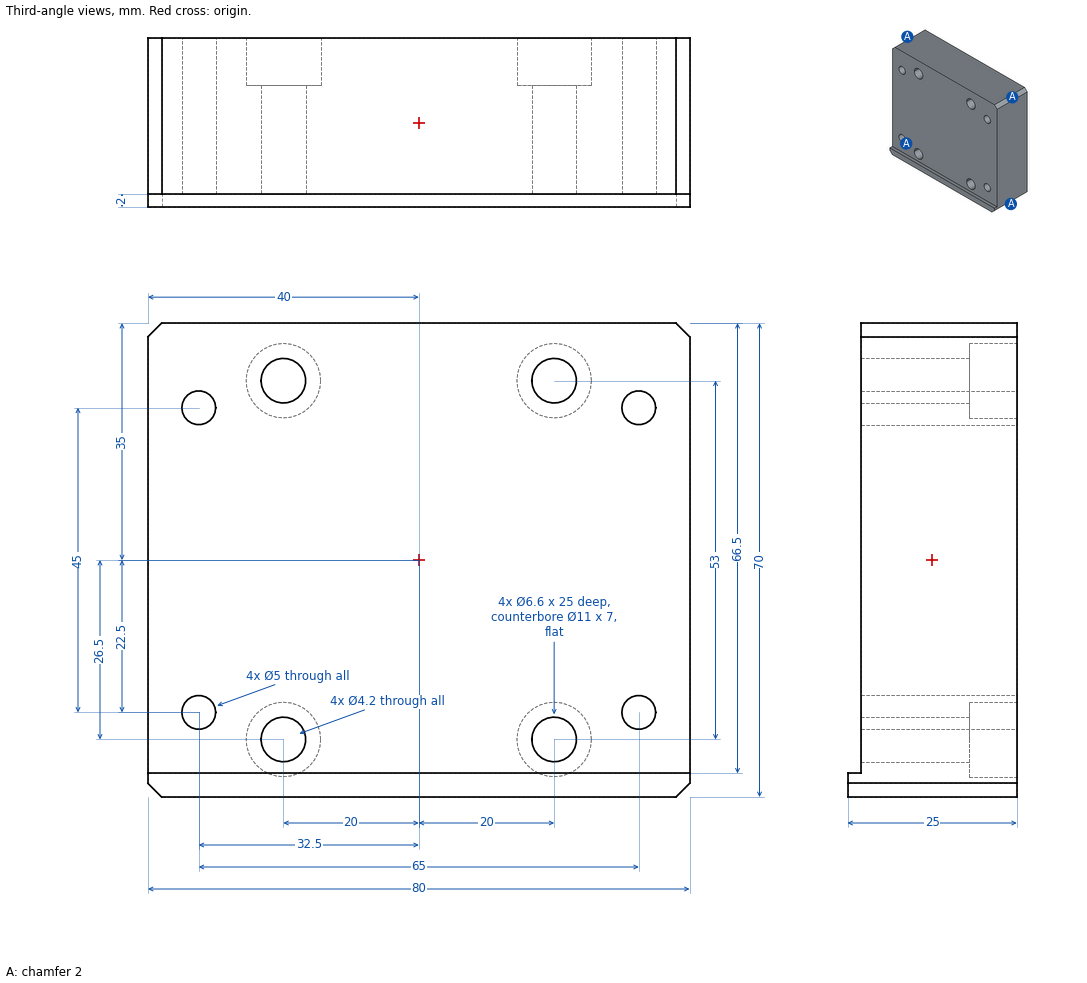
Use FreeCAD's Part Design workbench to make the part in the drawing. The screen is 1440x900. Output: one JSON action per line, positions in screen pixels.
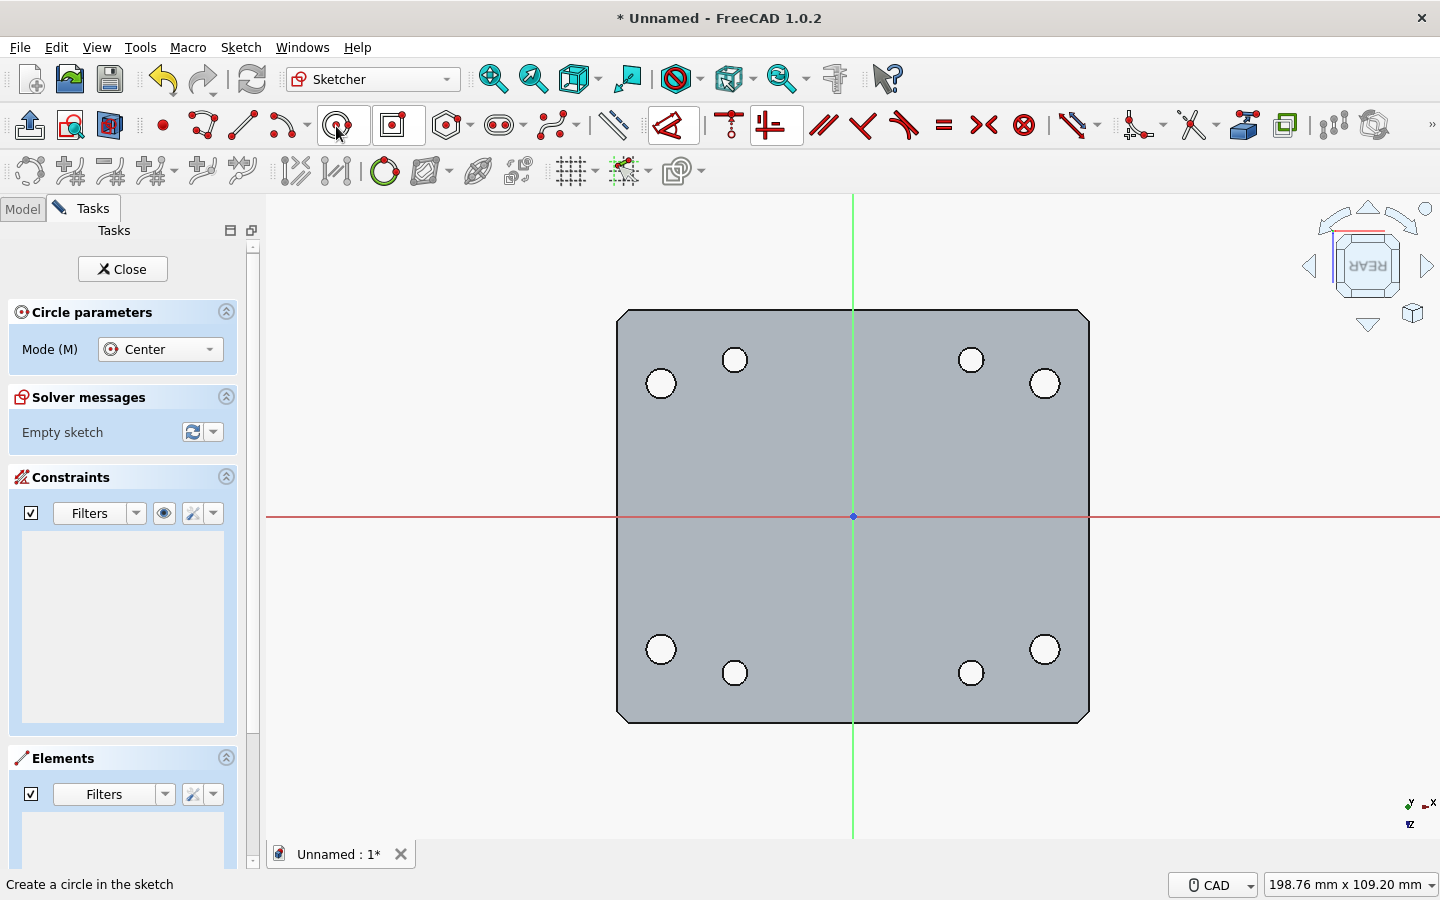
{"action": "left_click", "coordinate": [971, 360]}
{"action": "mouse_move", "coordinate": [985, 346]}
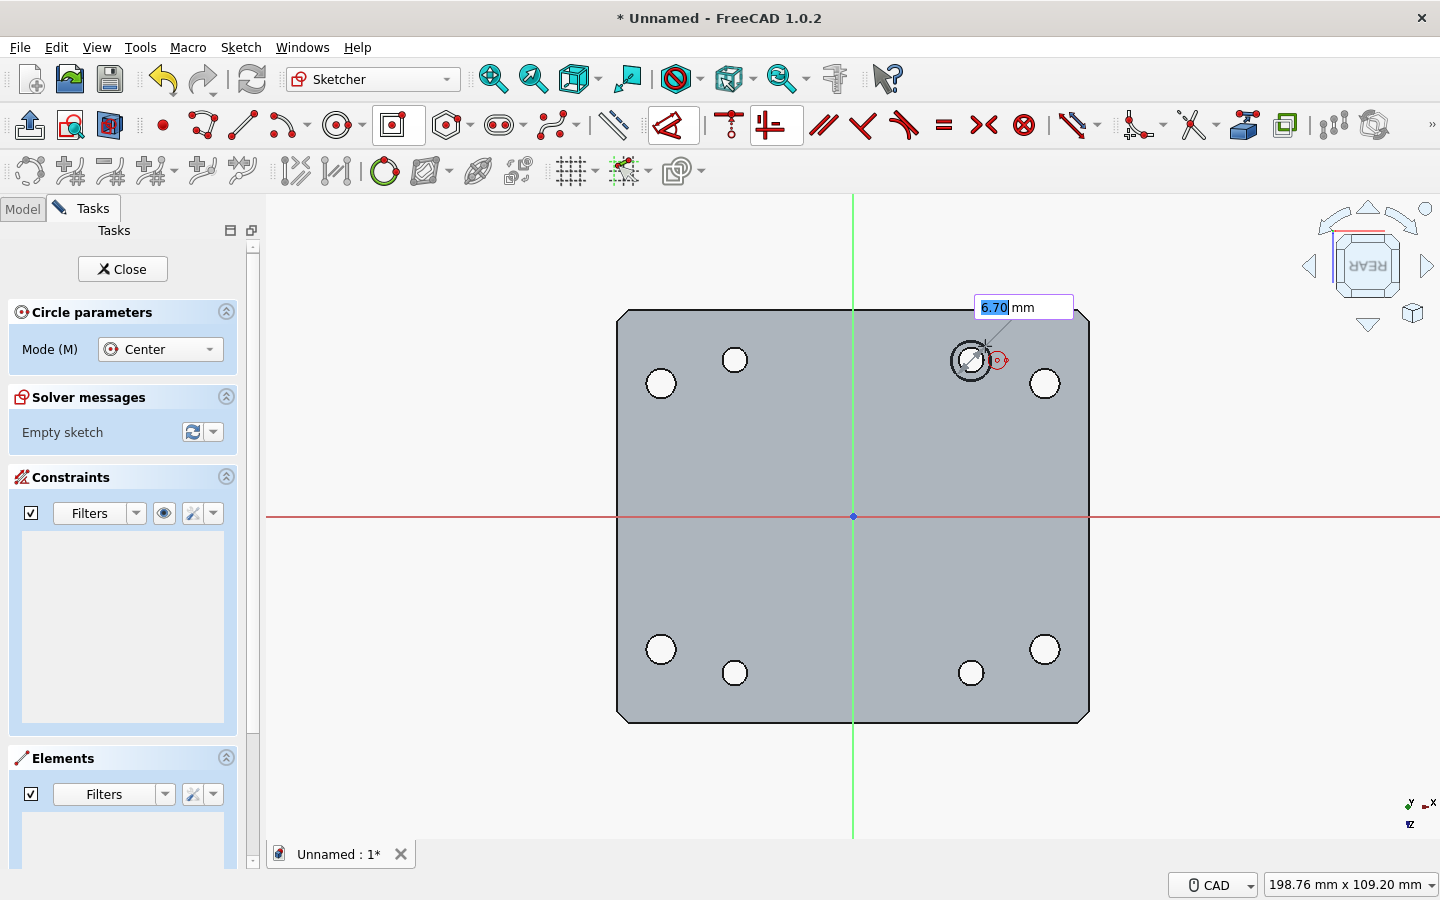
{"action": "type", "text": "6.6"}
{"action": "key", "text": "Return"}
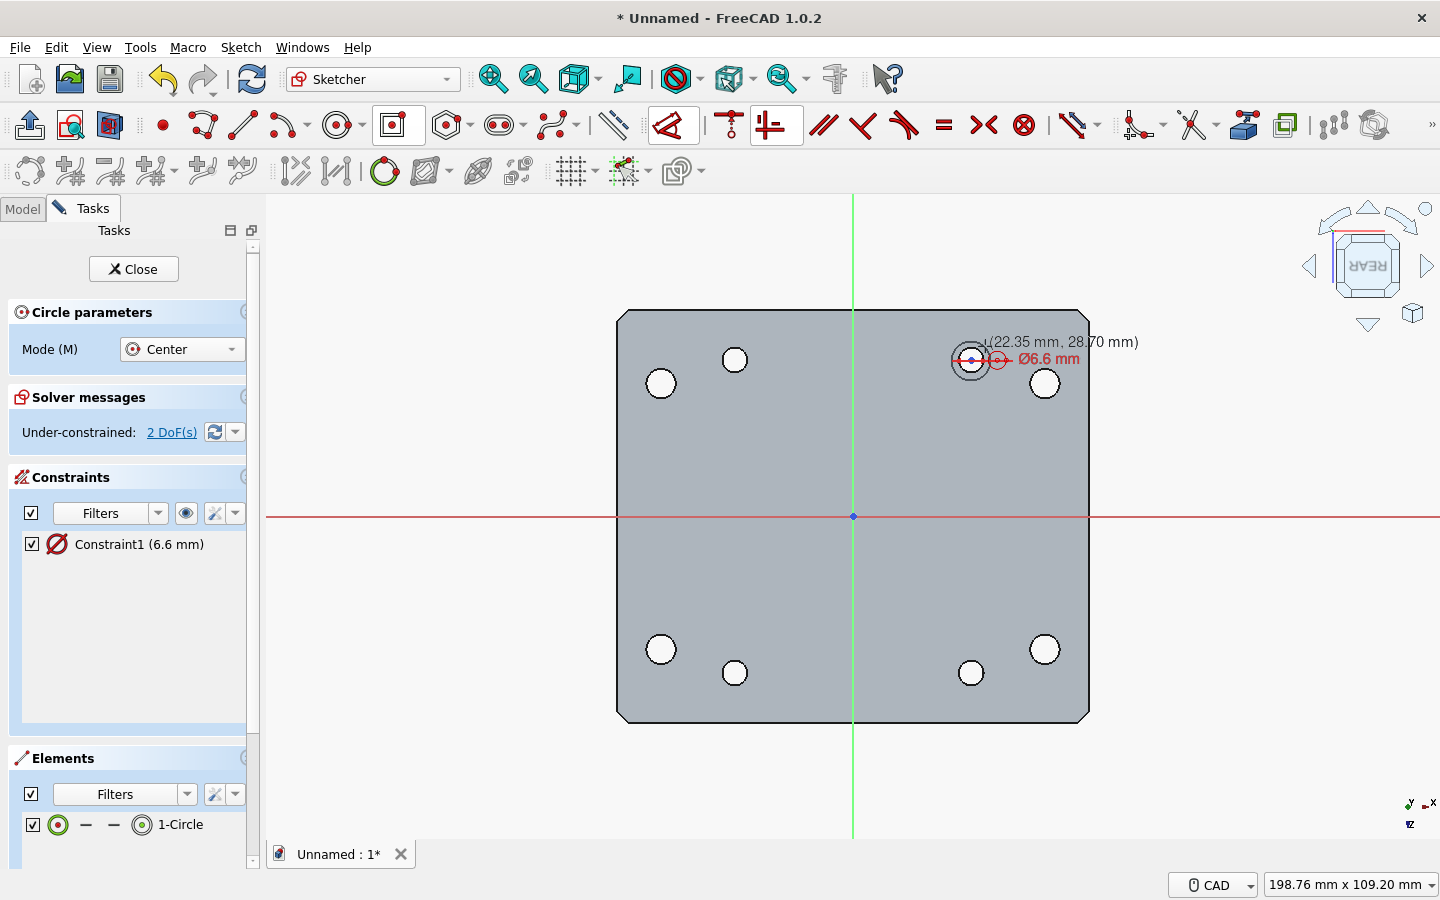
{"action": "left_click", "coordinate": [971, 673]}
{"action": "mouse_move", "coordinate": [985, 659]}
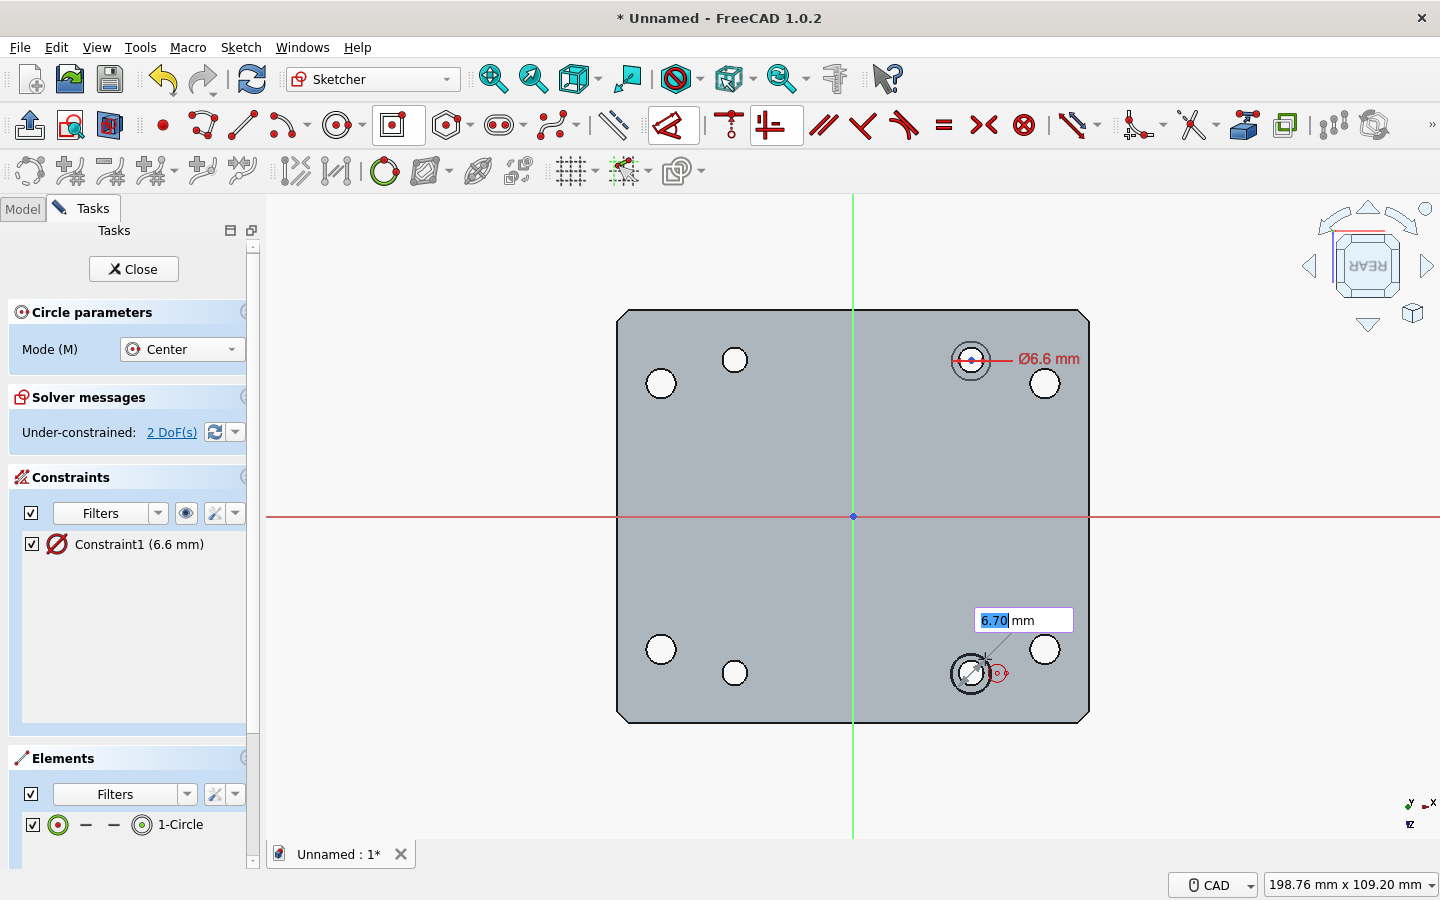
{"action": "type", "text": "6.6"}
{"action": "key", "text": "Return"}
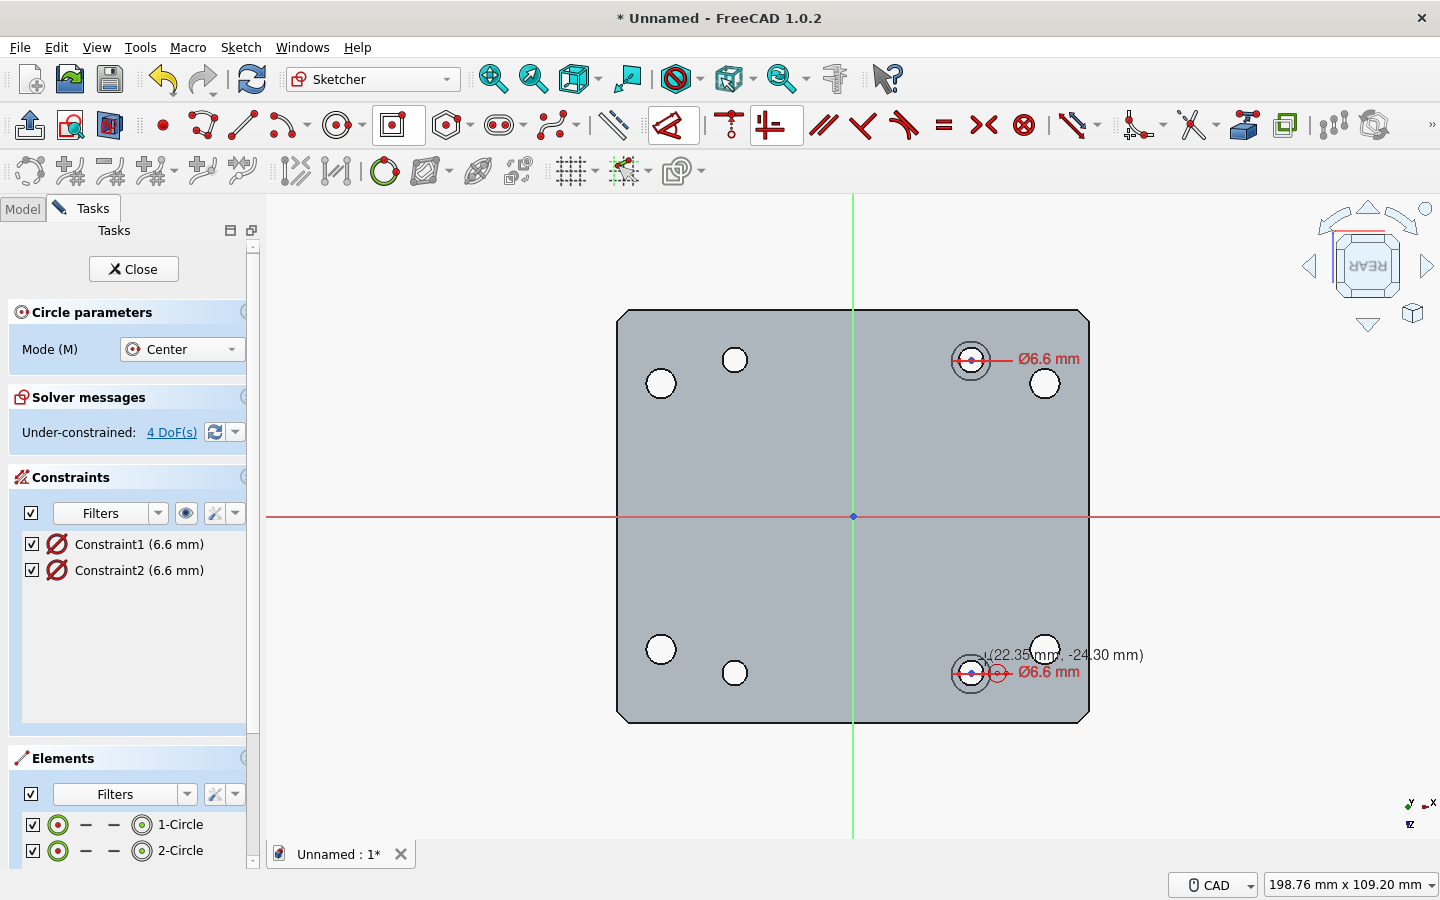
{"action": "left_click", "coordinate": [735, 673]}
{"action": "mouse_move", "coordinate": [749, 659]}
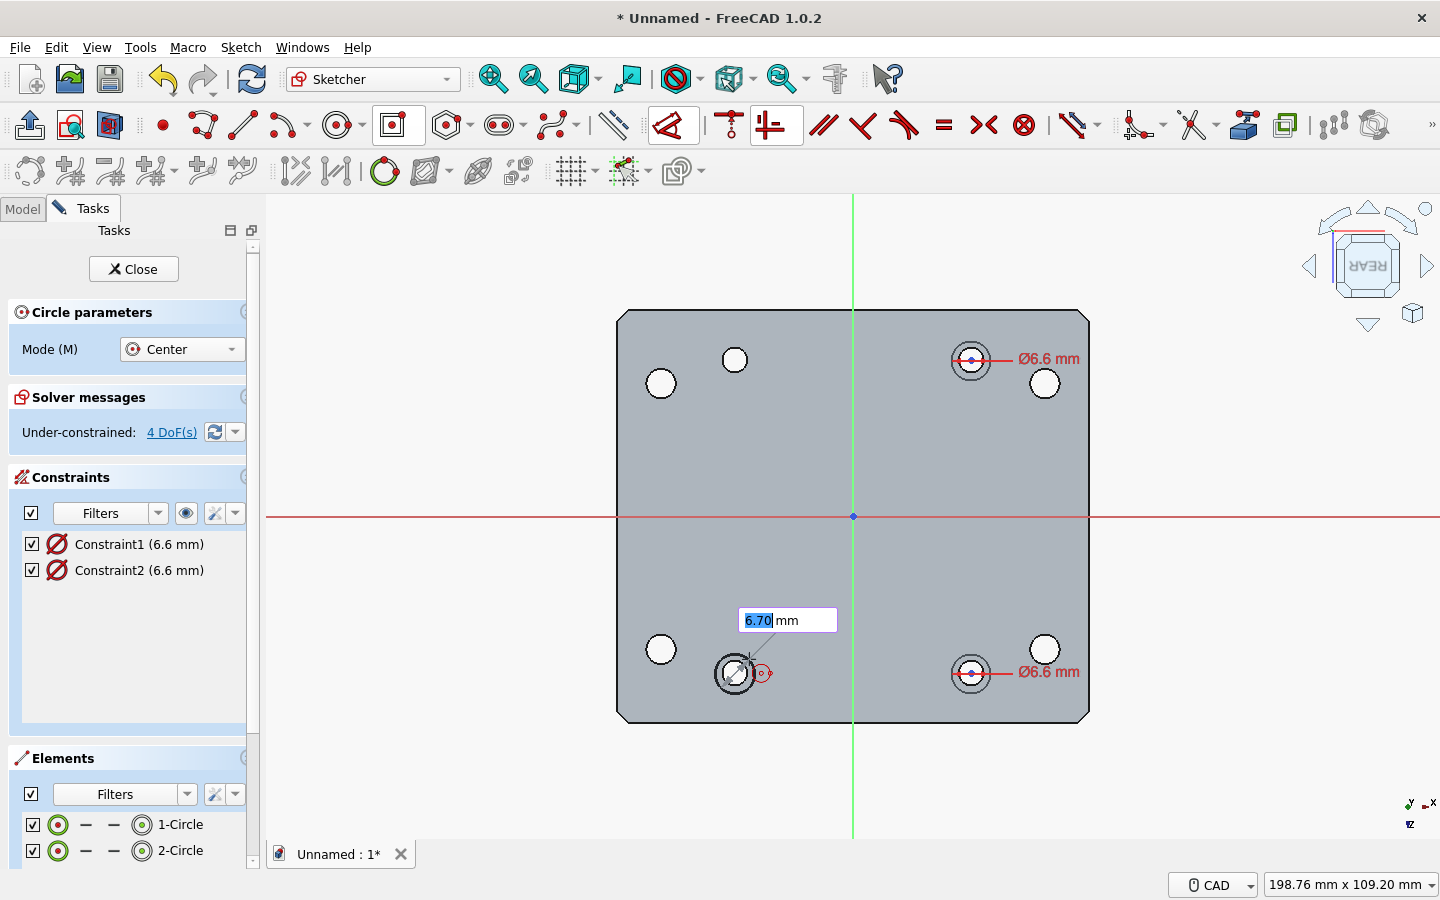
{"action": "type", "text": "6.6"}
{"action": "key", "text": "Return"}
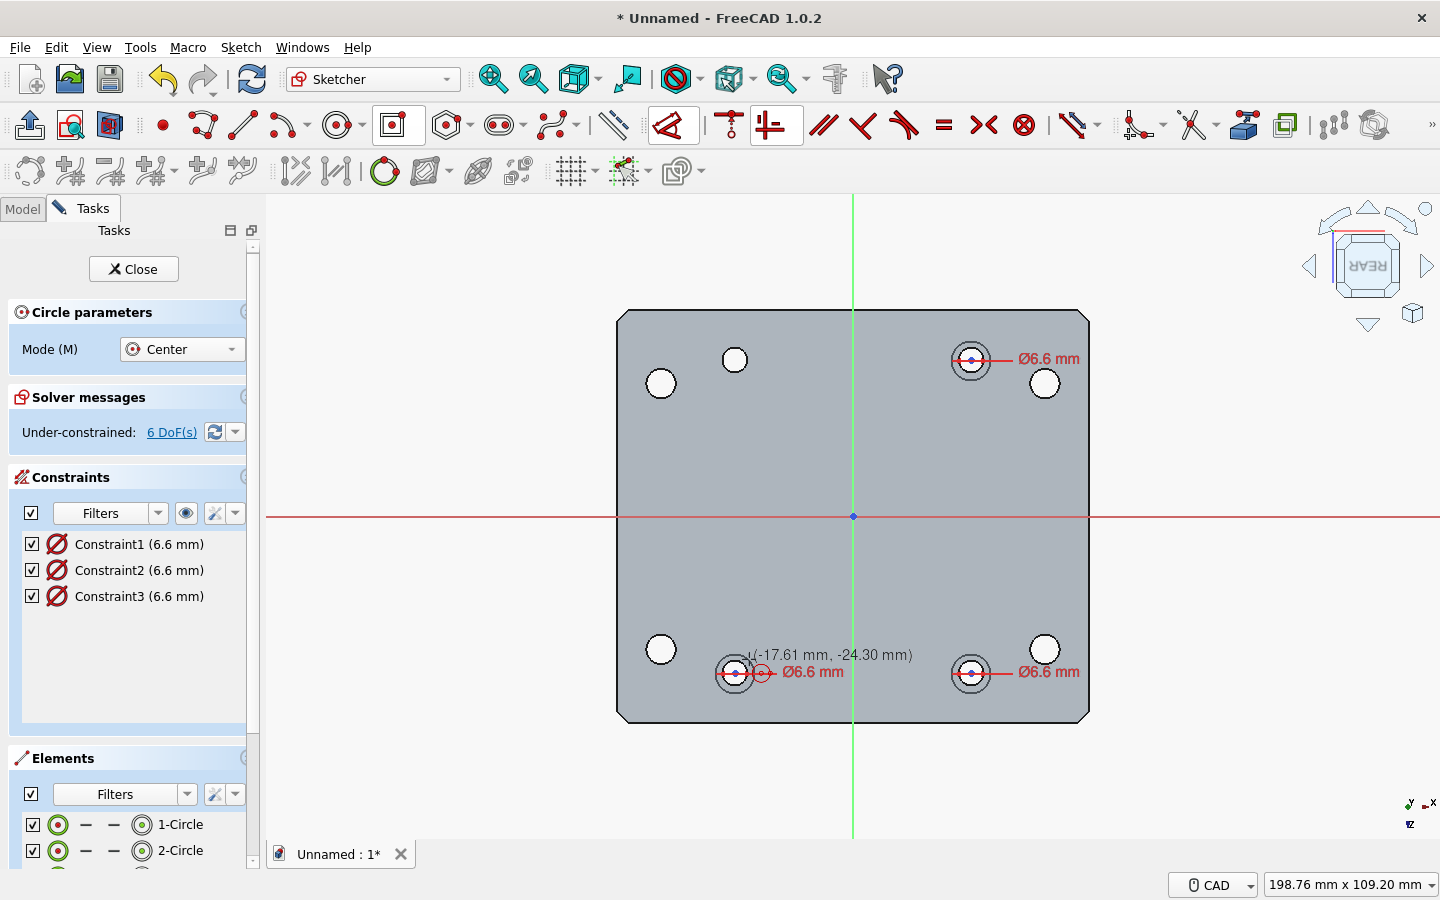
{"action": "left_click", "coordinate": [735, 360]}
{"action": "mouse_move", "coordinate": [749, 346]}